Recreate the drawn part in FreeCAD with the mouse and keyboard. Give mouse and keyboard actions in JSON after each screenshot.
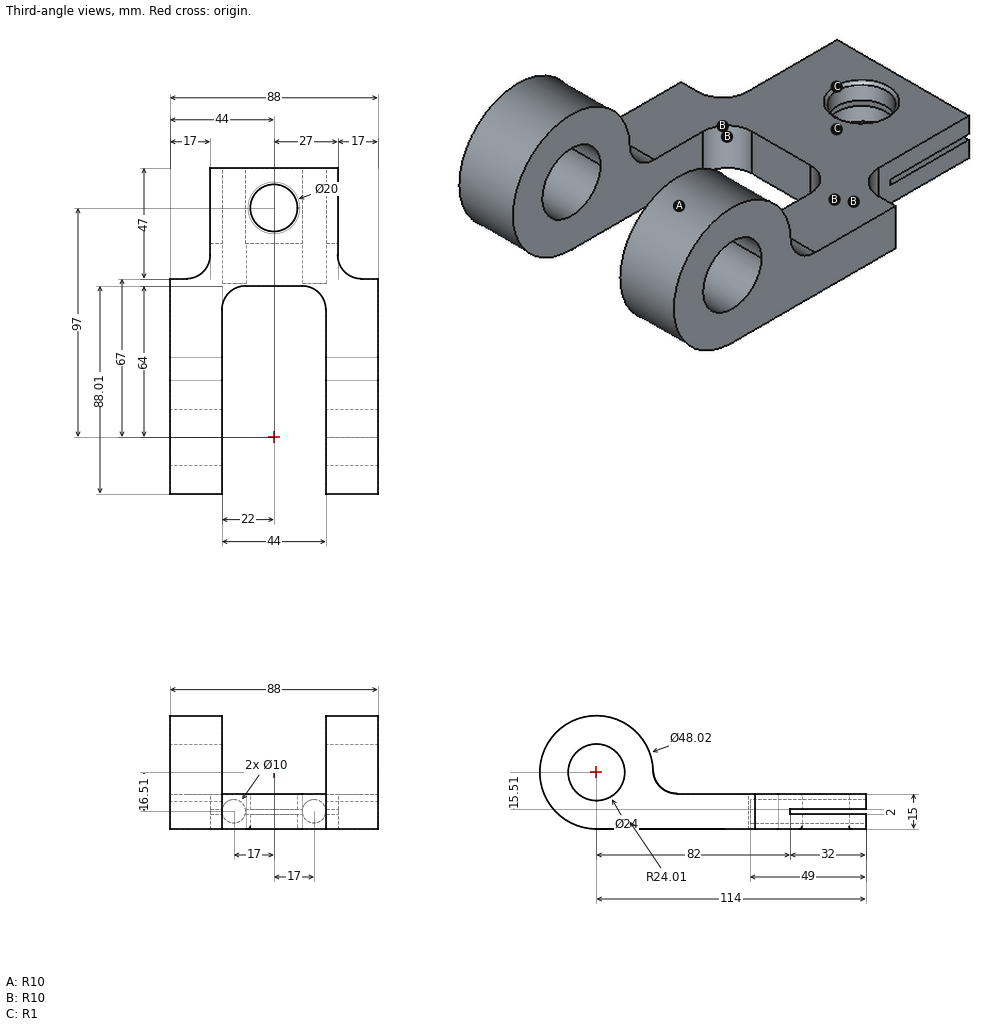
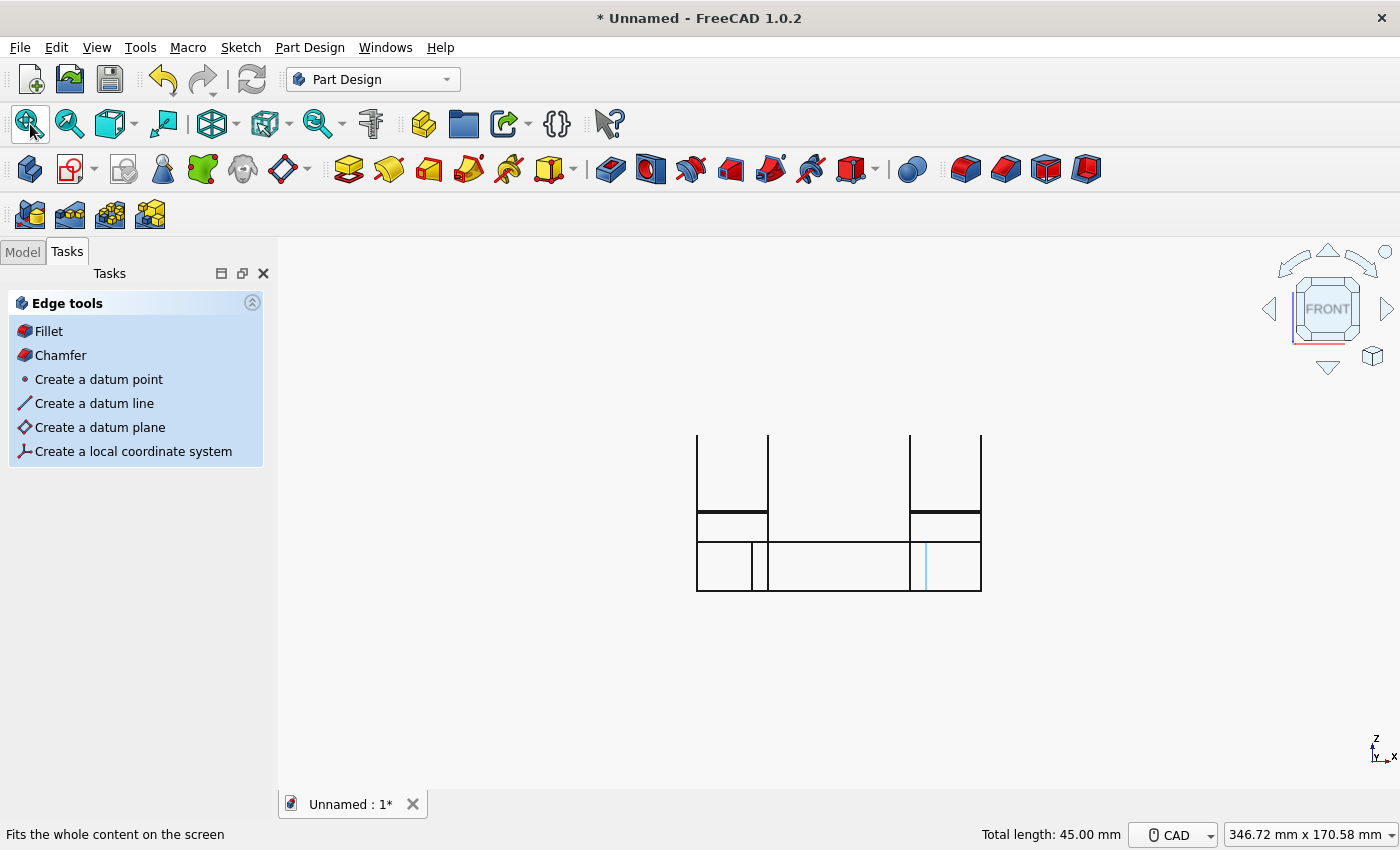
{"action": "left_click", "coordinate": [752, 565], "text": "ctrl"}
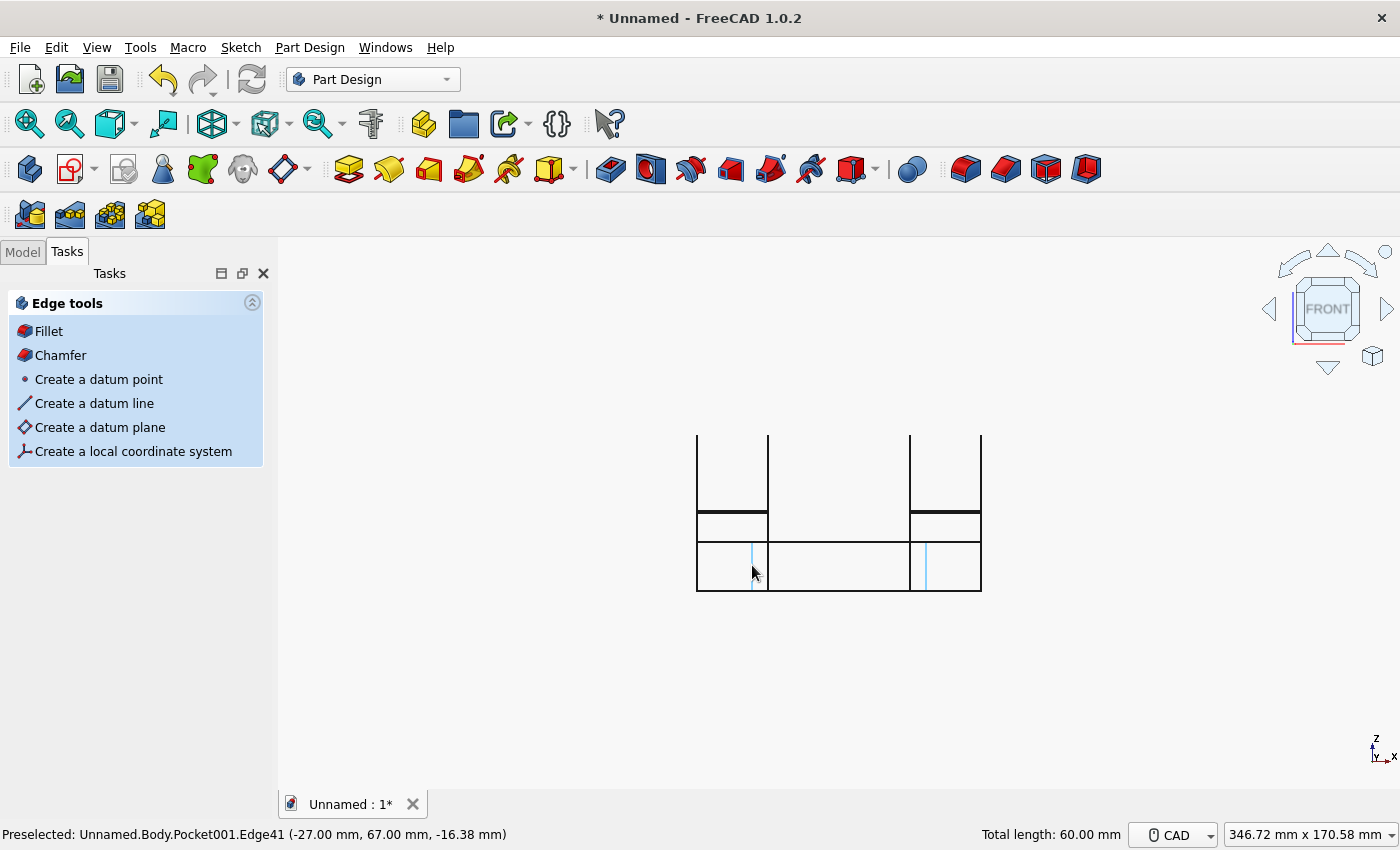
{"action": "key", "text": "v 1"}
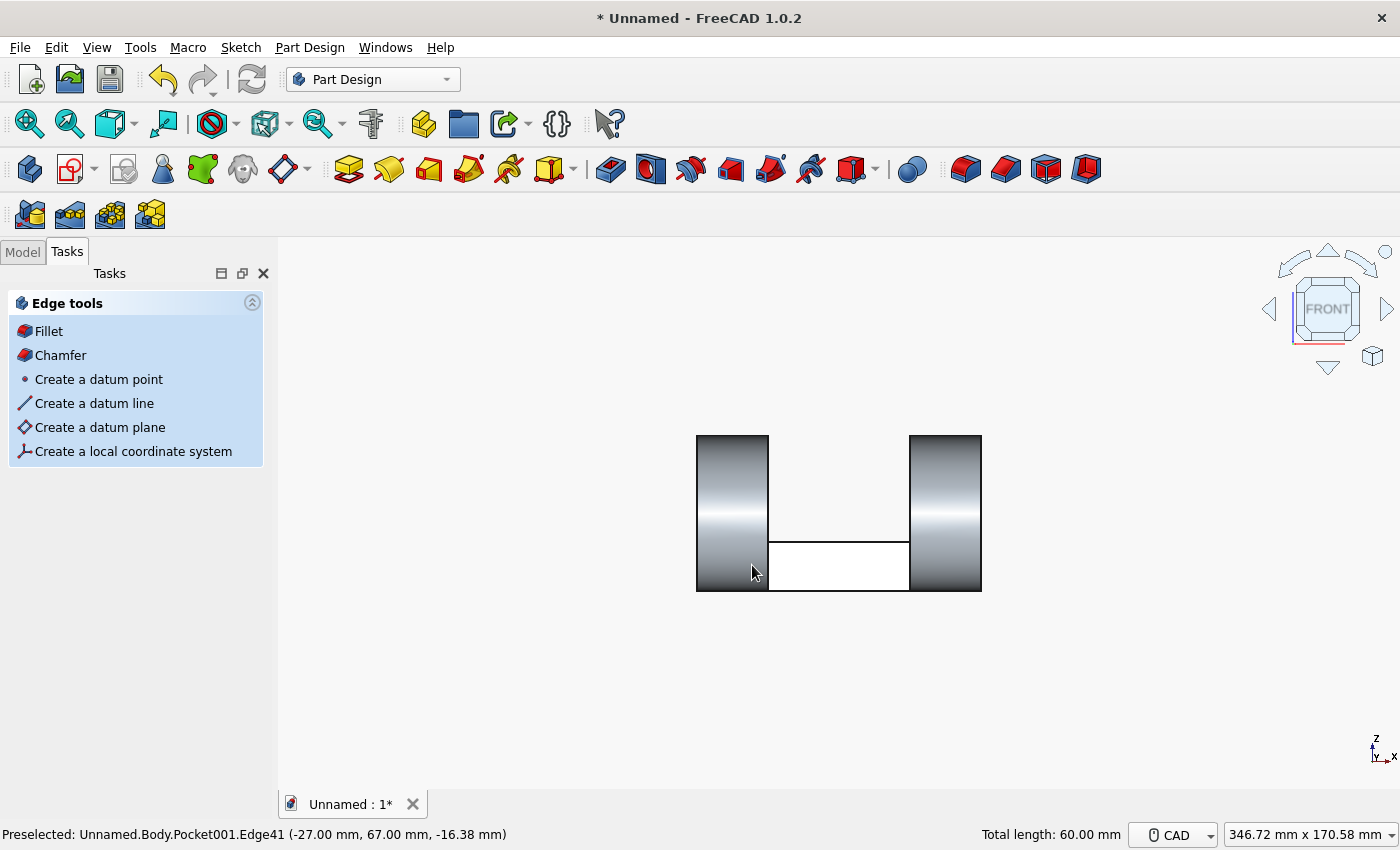
{"action": "left_click", "coordinate": [966, 170]}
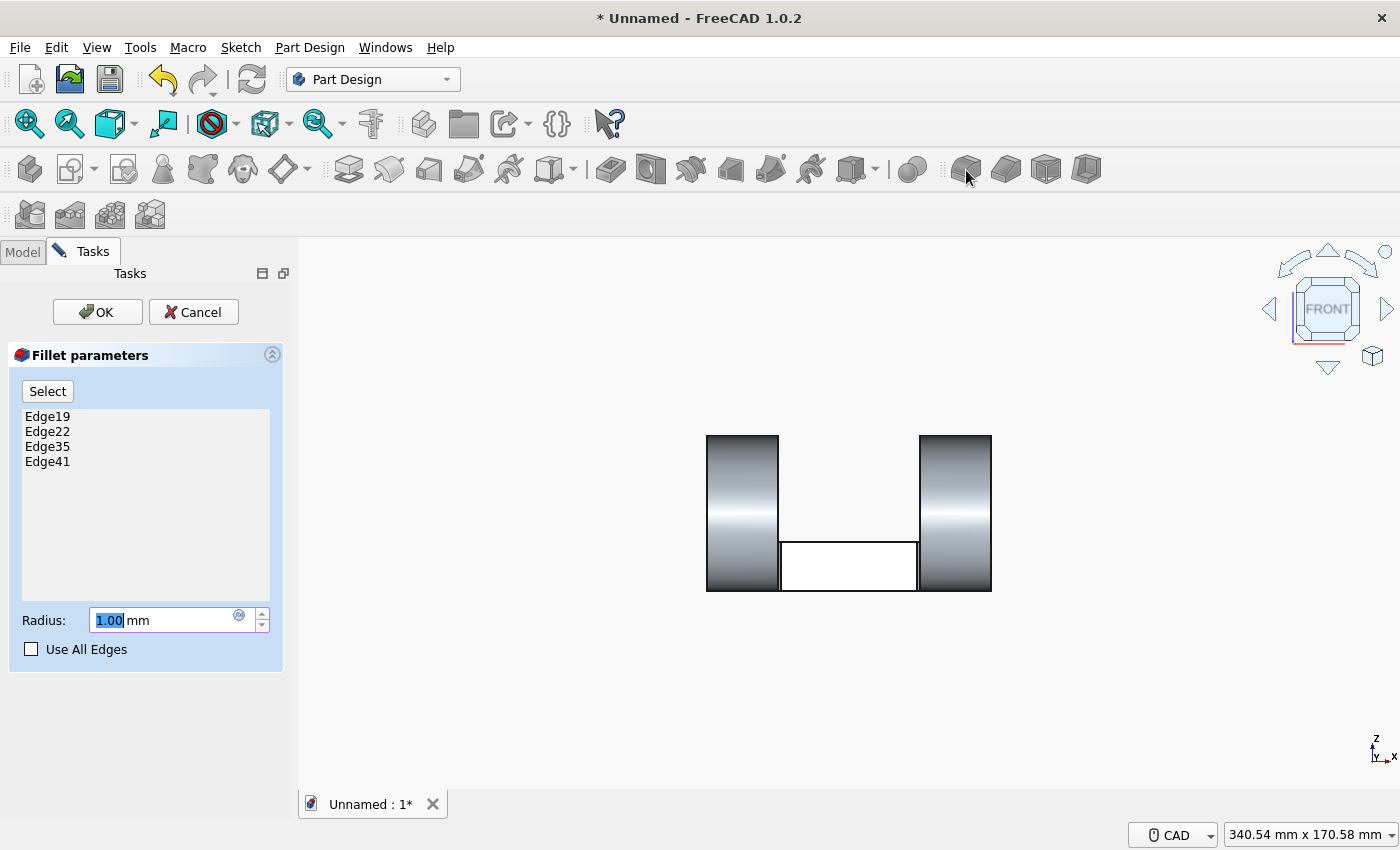
{"action": "type", "text": "10"}
{"action": "key", "text": "Tab"}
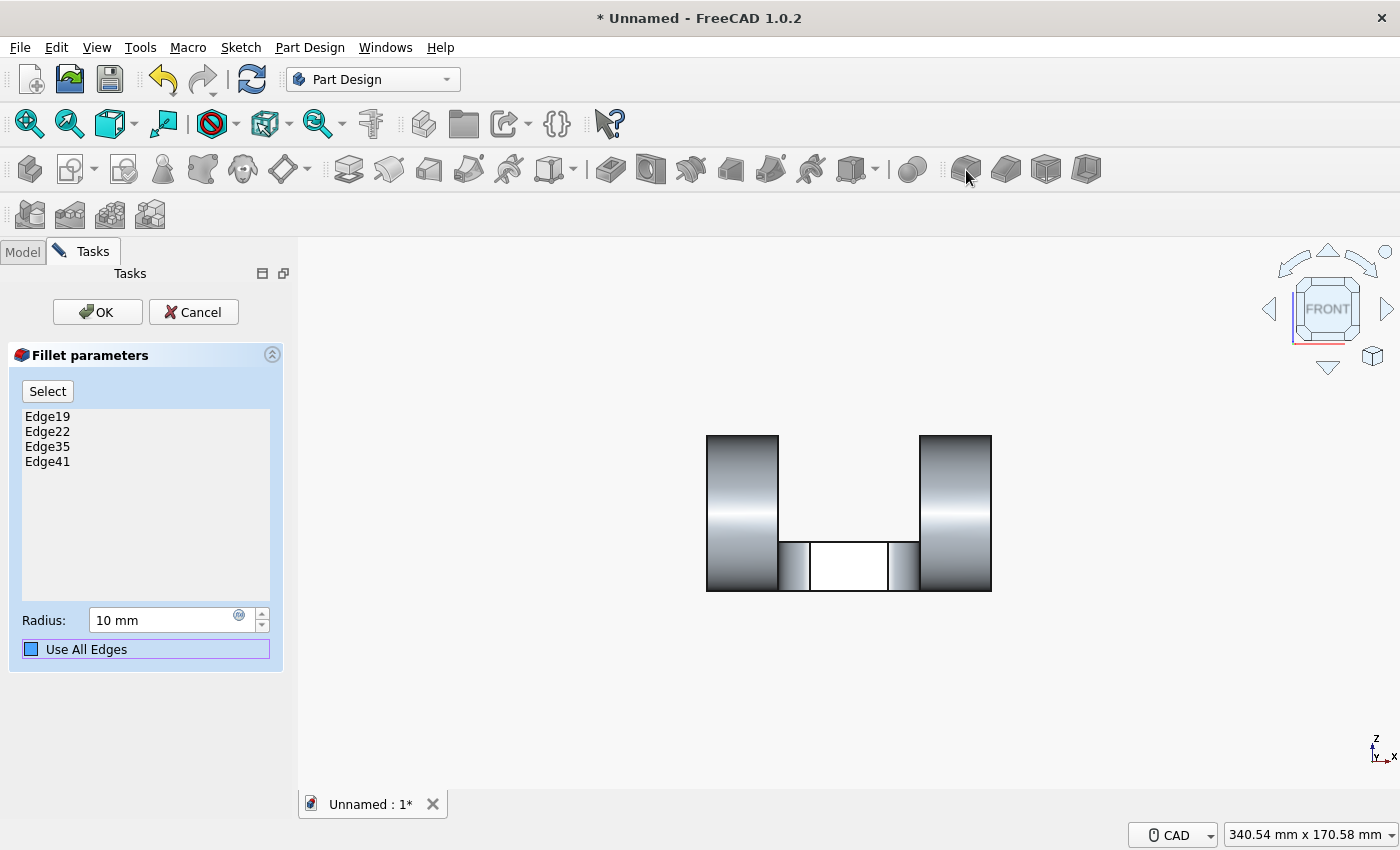
{"action": "left_click", "coordinate": [98, 312]}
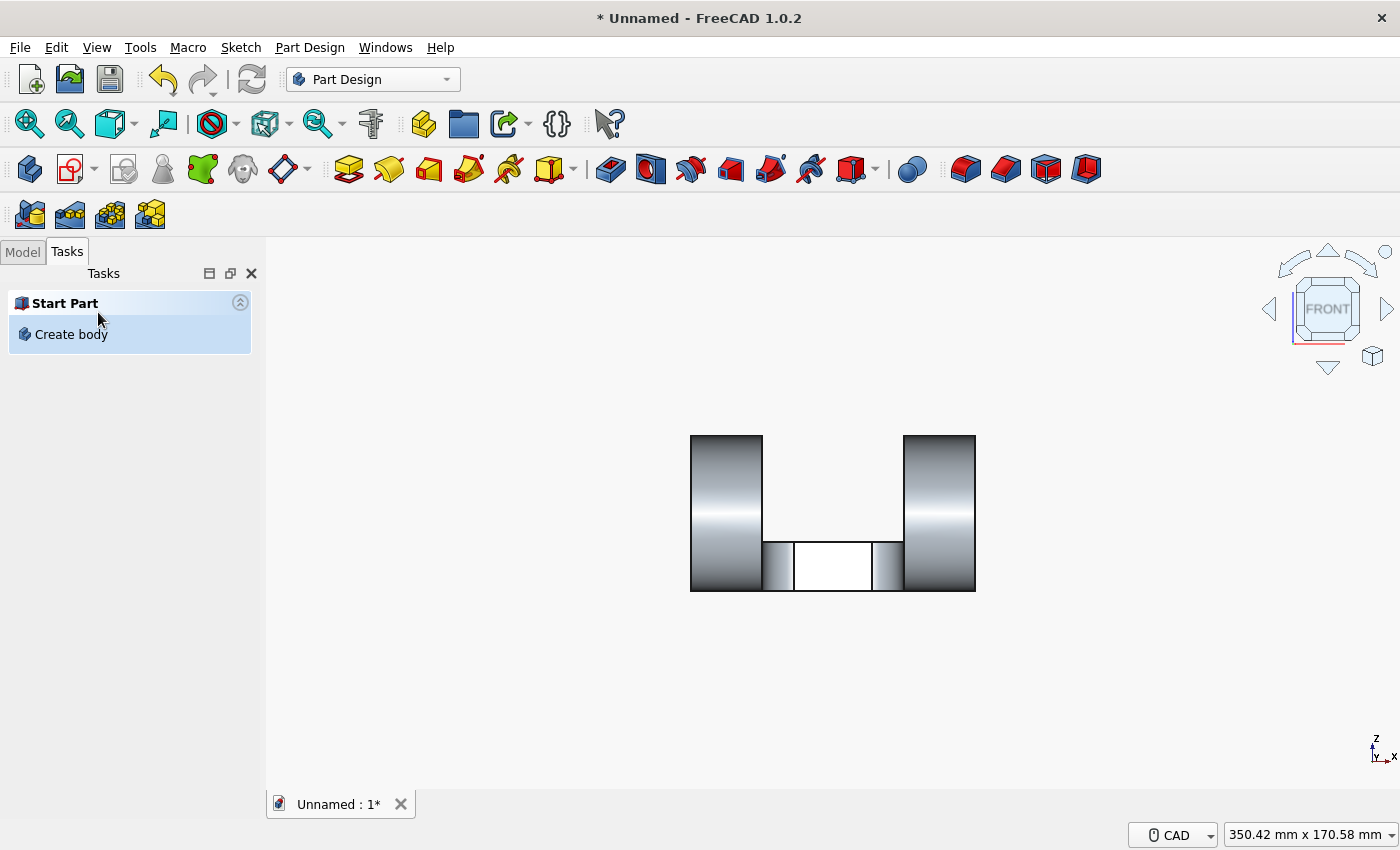
{"action": "left_click", "coordinate": [30, 124]}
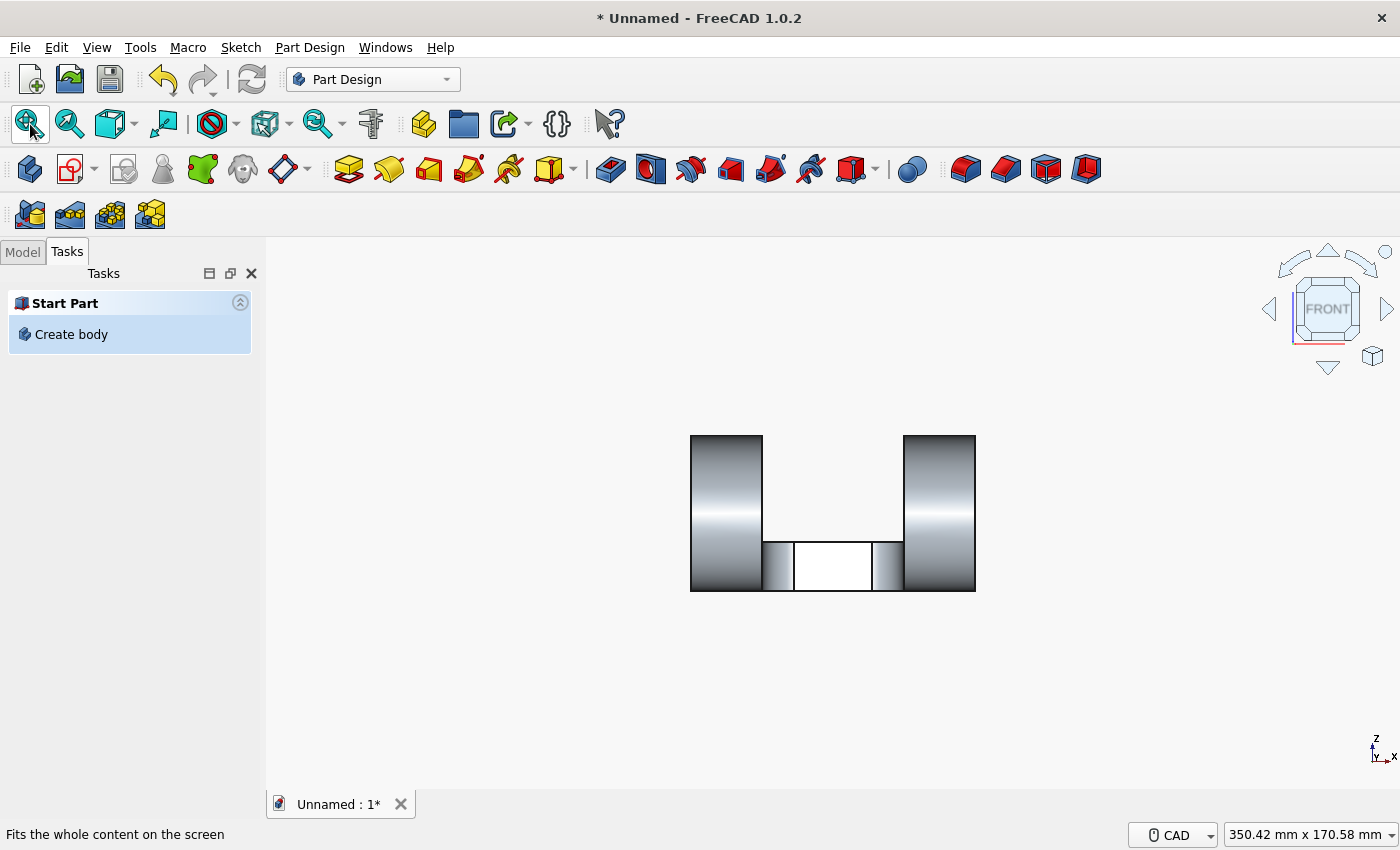
{"action": "left_click", "coordinate": [70, 170]}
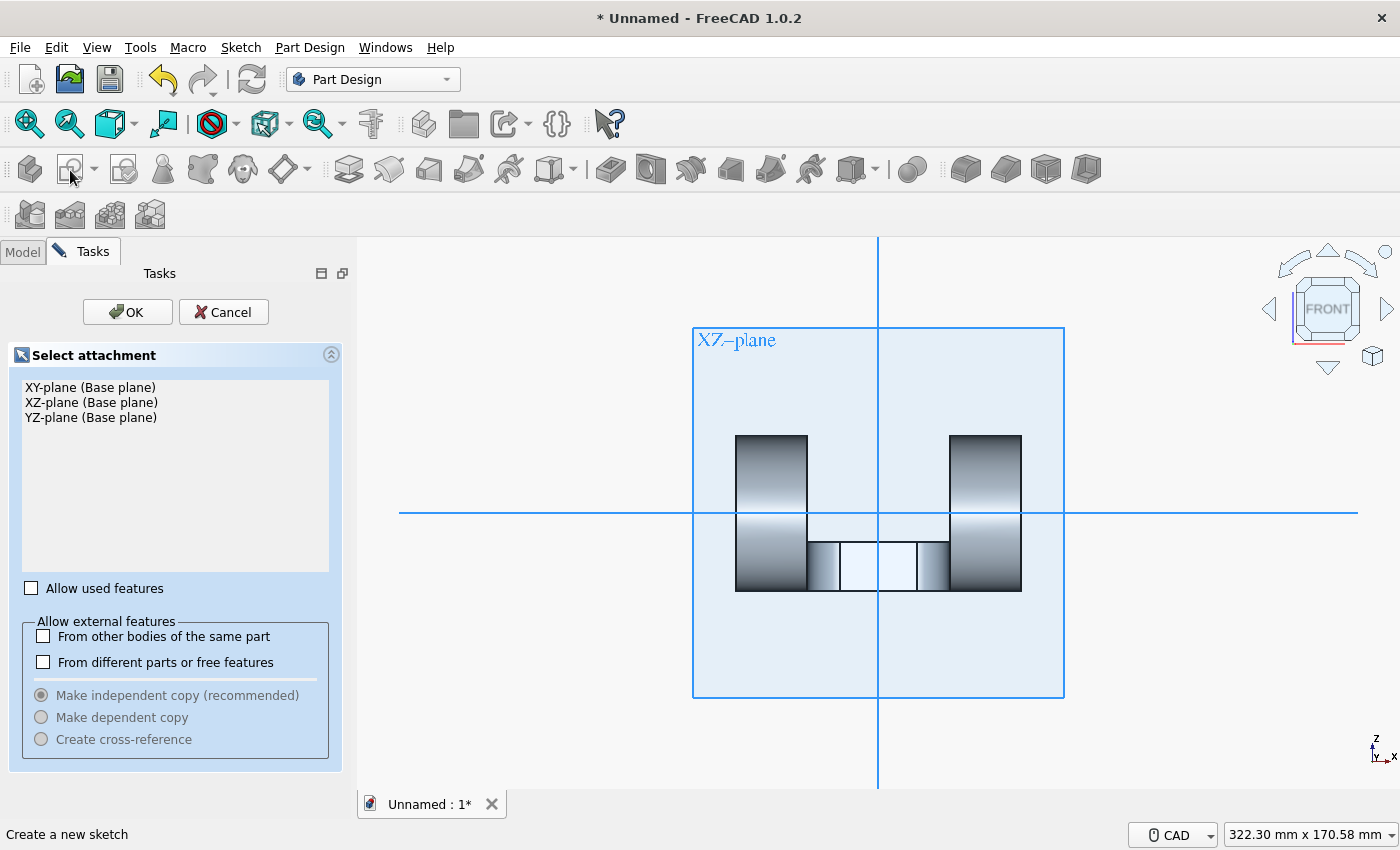
{"action": "left_click", "coordinate": [82, 418]}